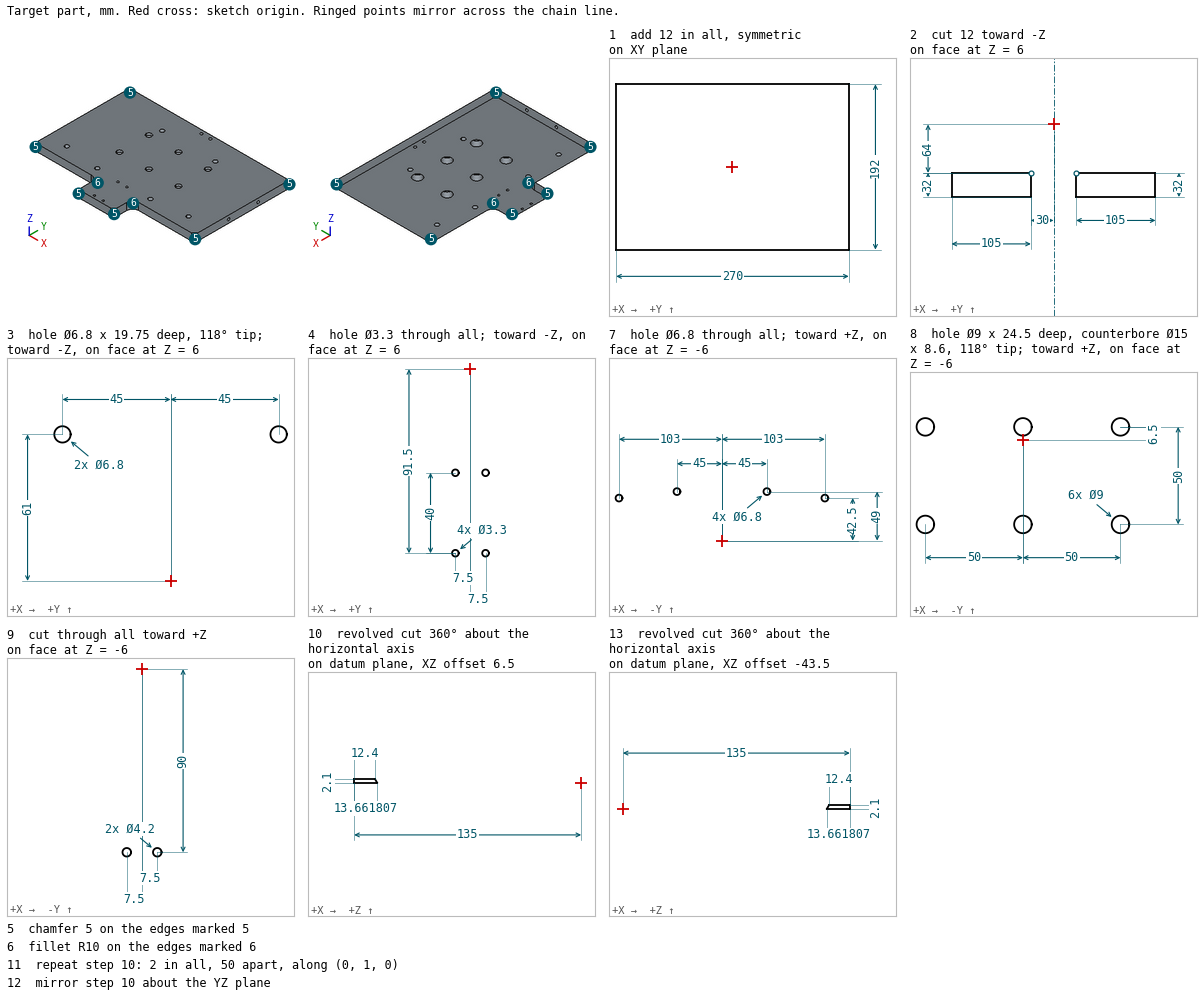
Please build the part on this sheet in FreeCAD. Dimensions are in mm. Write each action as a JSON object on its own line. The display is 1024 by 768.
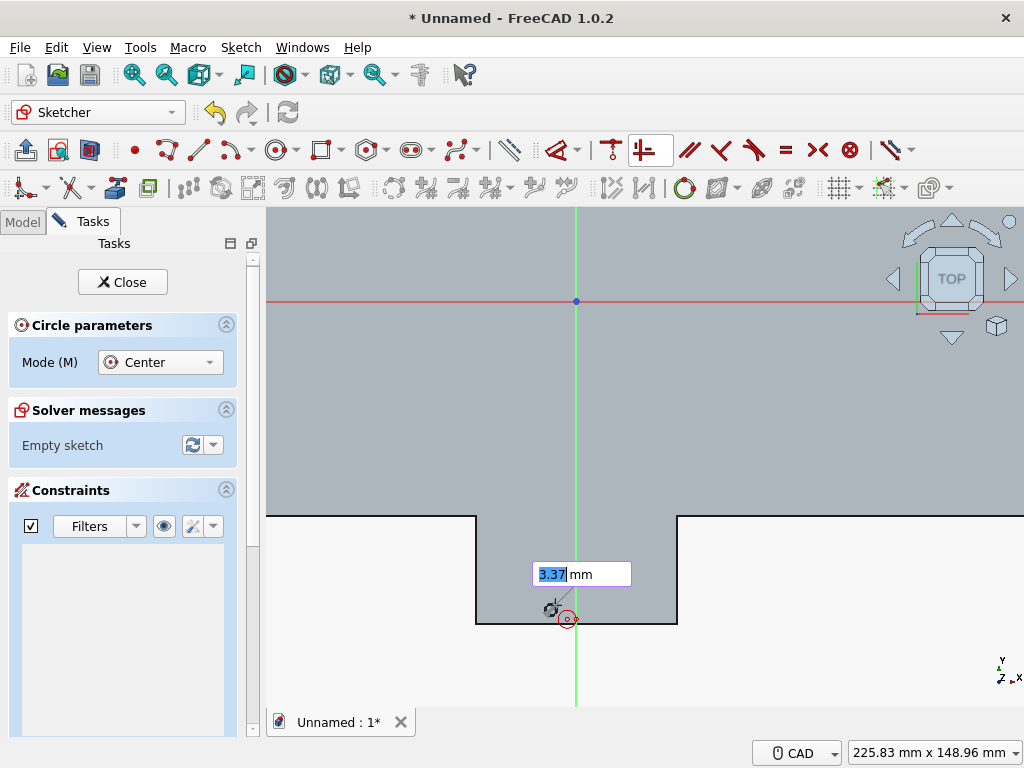
{"action": "type", "text": "3.3"}
{"action": "key", "text": "Return"}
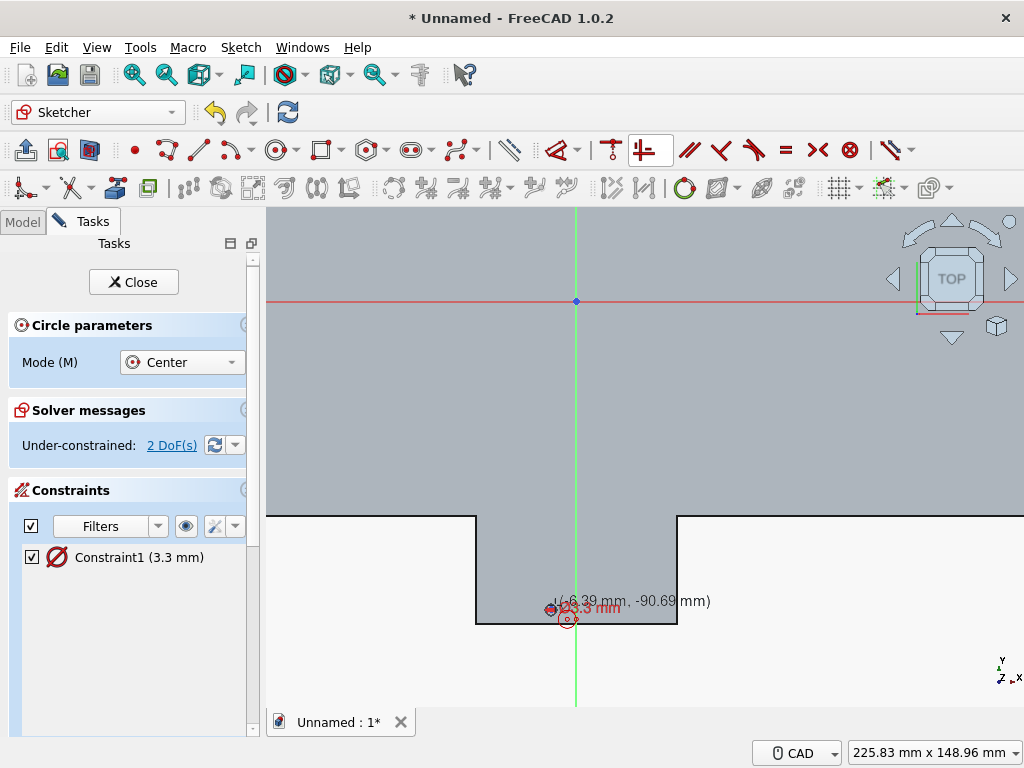
{"action": "scroll", "coordinate": [602, 609], "scroll_direction": "up", "scroll_amount": 8}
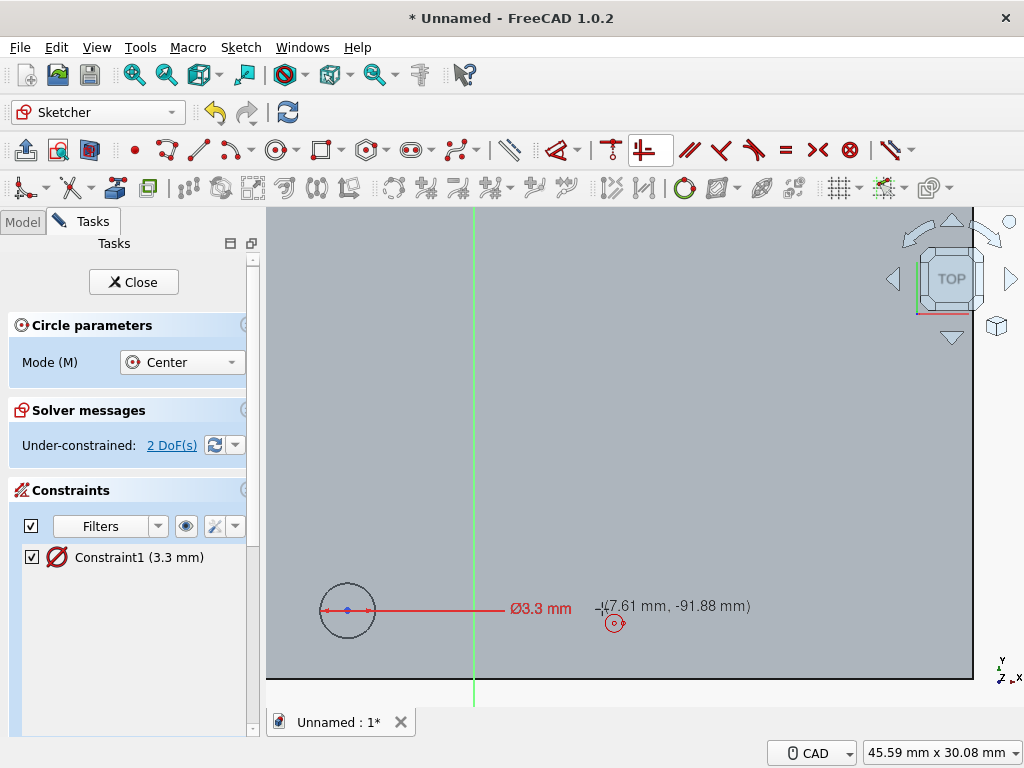
{"action": "scroll", "coordinate": [602, 609], "scroll_direction": "down", "scroll_amount": 8}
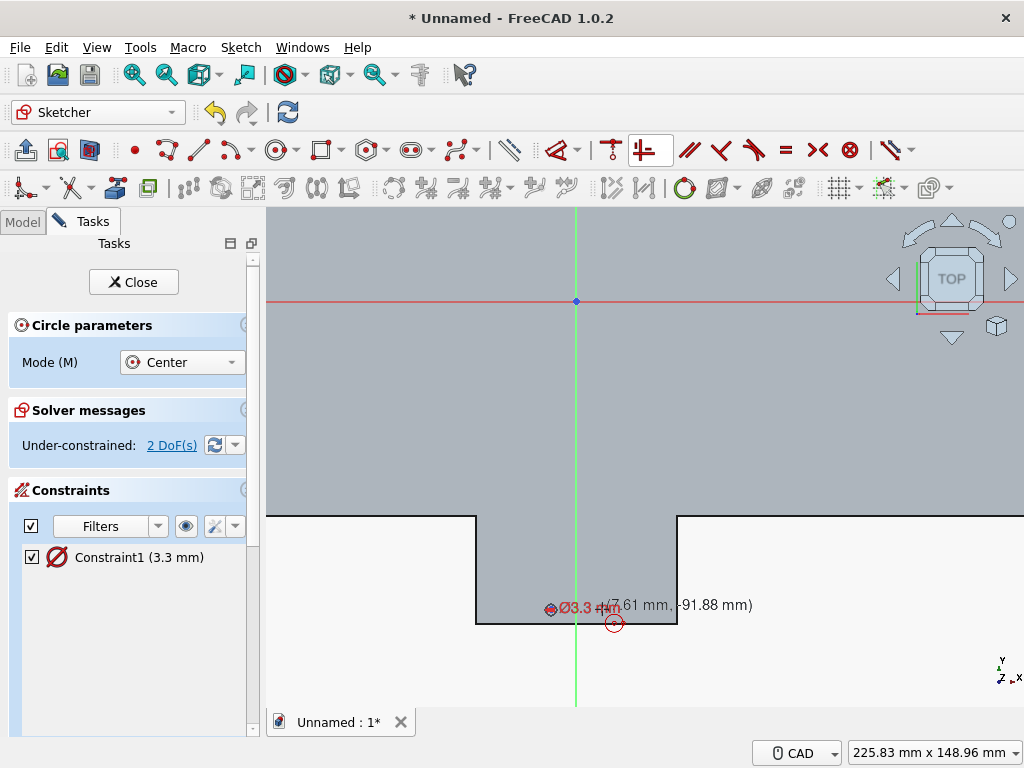
{"action": "left_click", "coordinate": [602, 609]}
{"action": "mouse_move", "coordinate": [606, 605]}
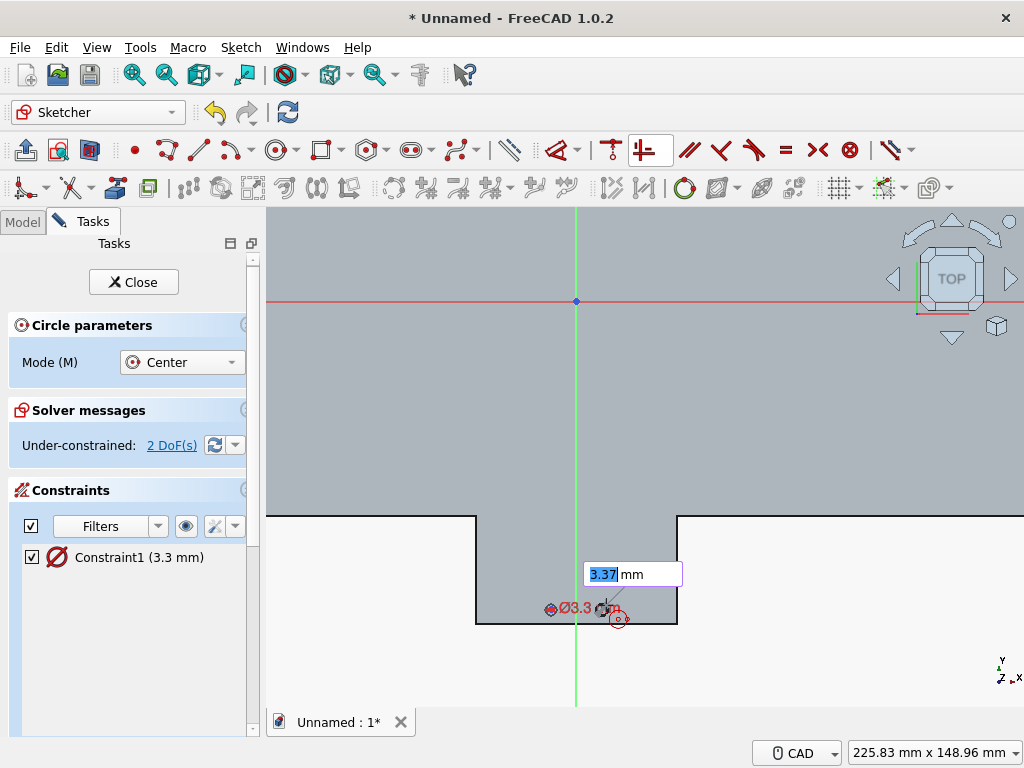
{"action": "type", "text": "3.3"}
{"action": "key", "text": "Return"}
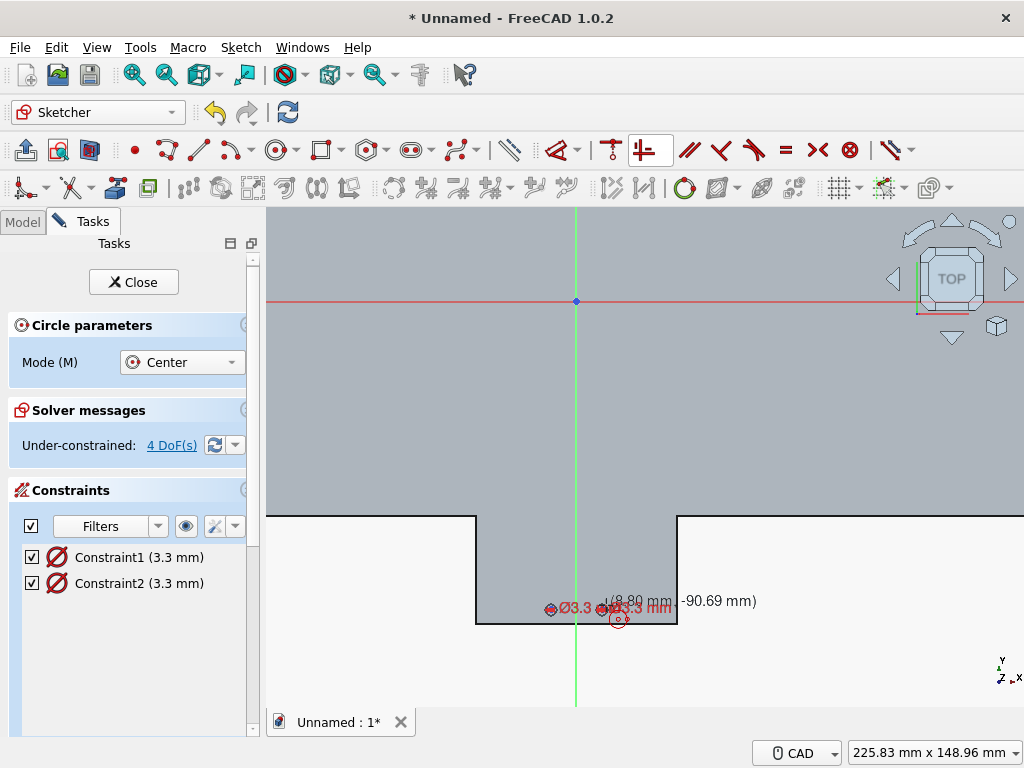
{"action": "scroll", "coordinate": [551, 474], "scroll_direction": "up", "scroll_amount": 8}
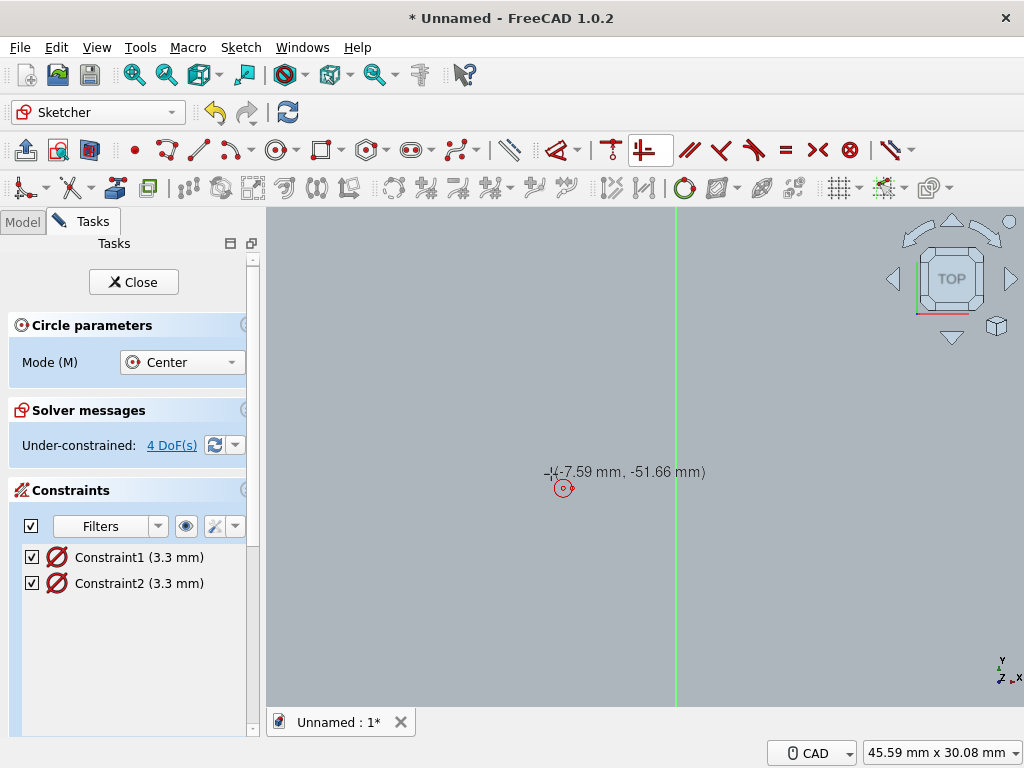
{"action": "scroll", "coordinate": [551, 473], "scroll_direction": "down", "scroll_amount": 8}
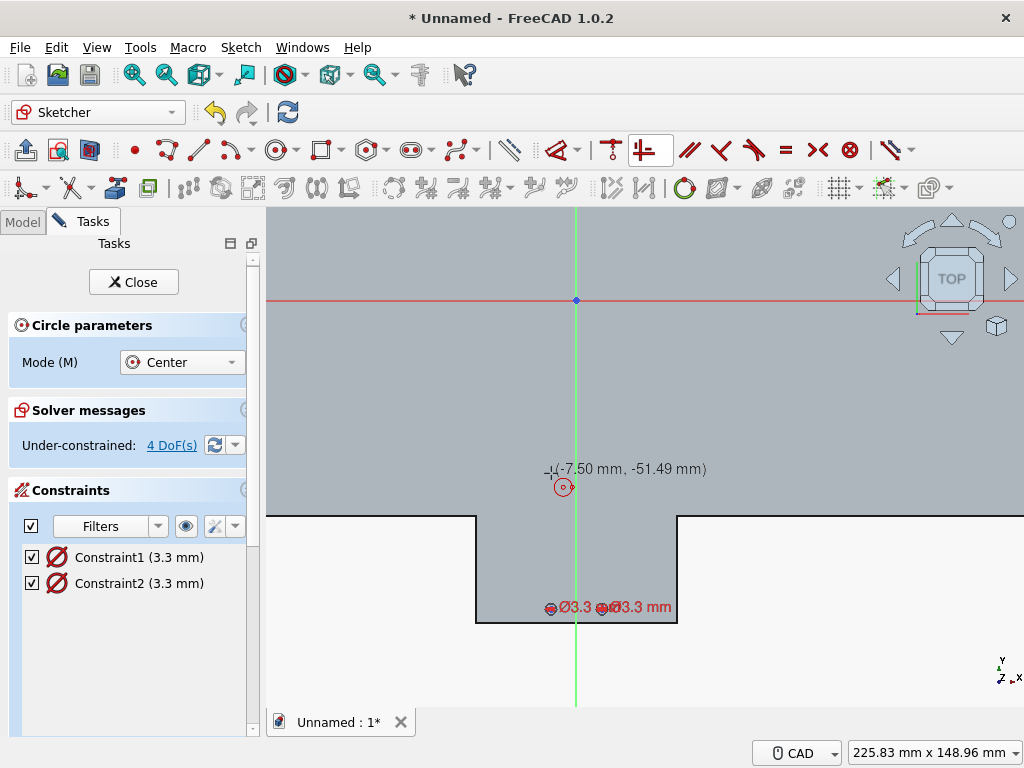
{"action": "left_click", "coordinate": [551, 474]}
{"action": "mouse_move", "coordinate": [555, 470]}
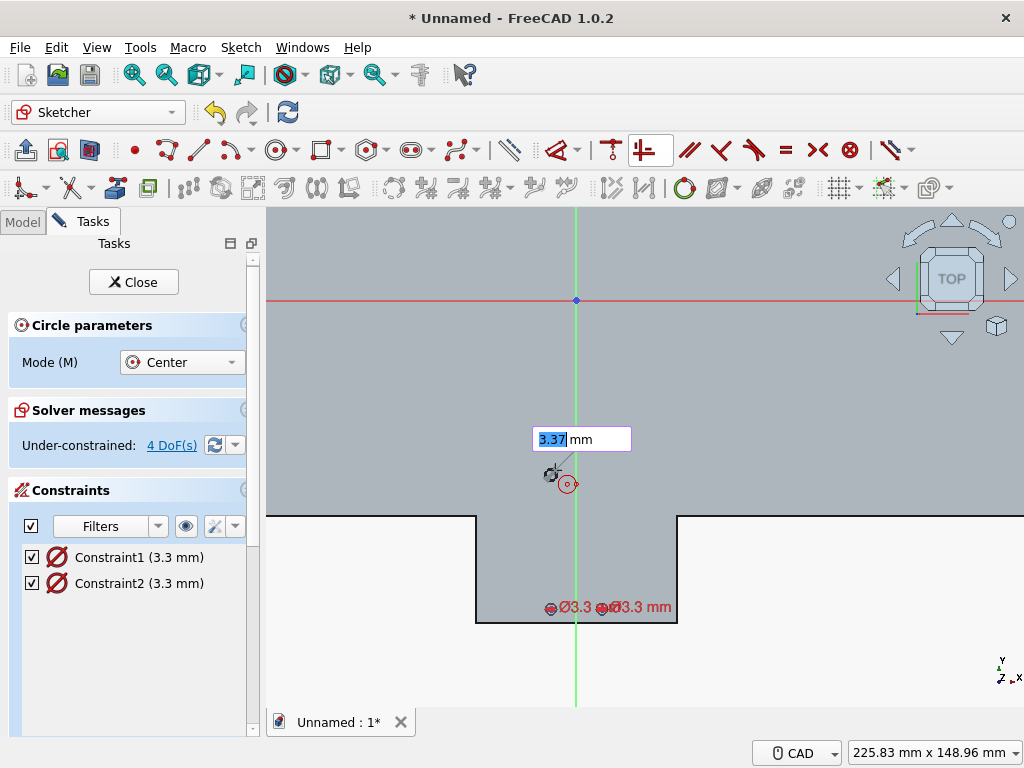
{"action": "type", "text": "3.3"}
{"action": "key", "text": "Return"}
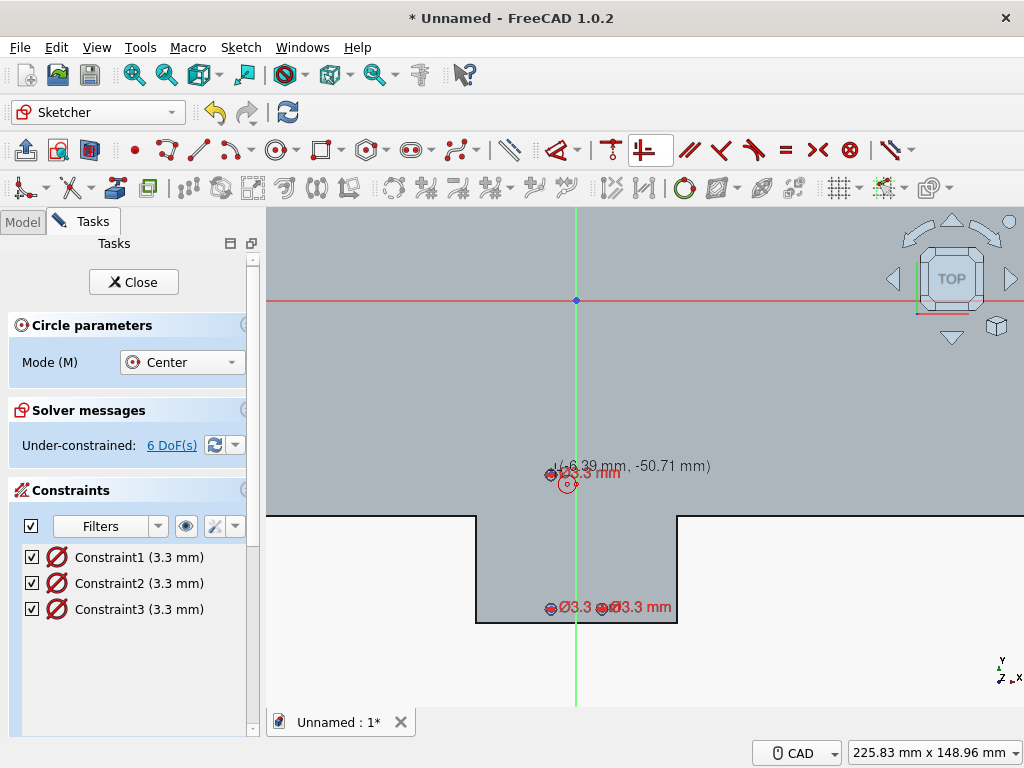
{"action": "scroll", "coordinate": [602, 474], "scroll_direction": "up", "scroll_amount": 8}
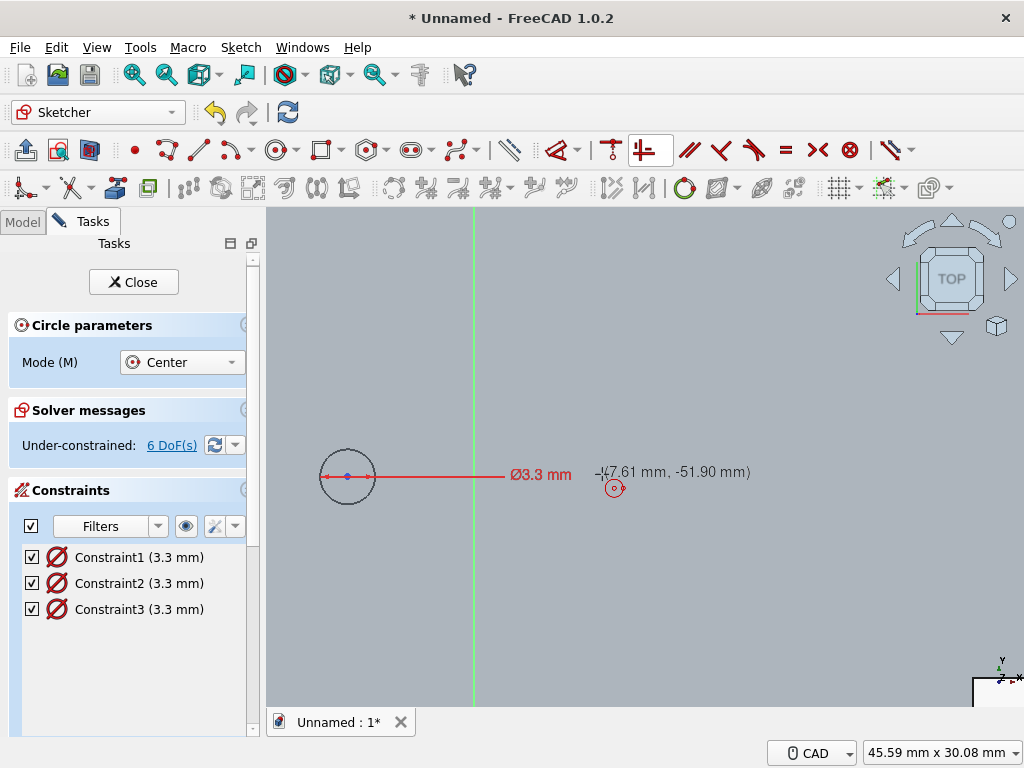
{"action": "scroll", "coordinate": [602, 474], "scroll_direction": "down", "scroll_amount": 8}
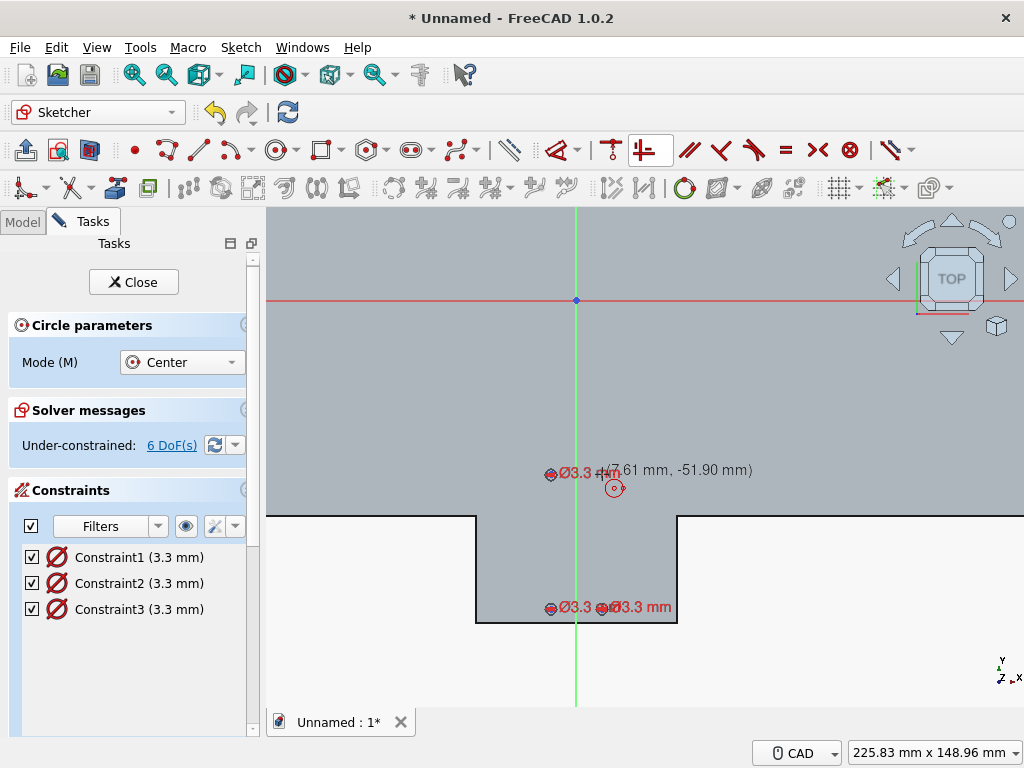
{"action": "left_click", "coordinate": [602, 474]}
{"action": "mouse_move", "coordinate": [606, 470]}